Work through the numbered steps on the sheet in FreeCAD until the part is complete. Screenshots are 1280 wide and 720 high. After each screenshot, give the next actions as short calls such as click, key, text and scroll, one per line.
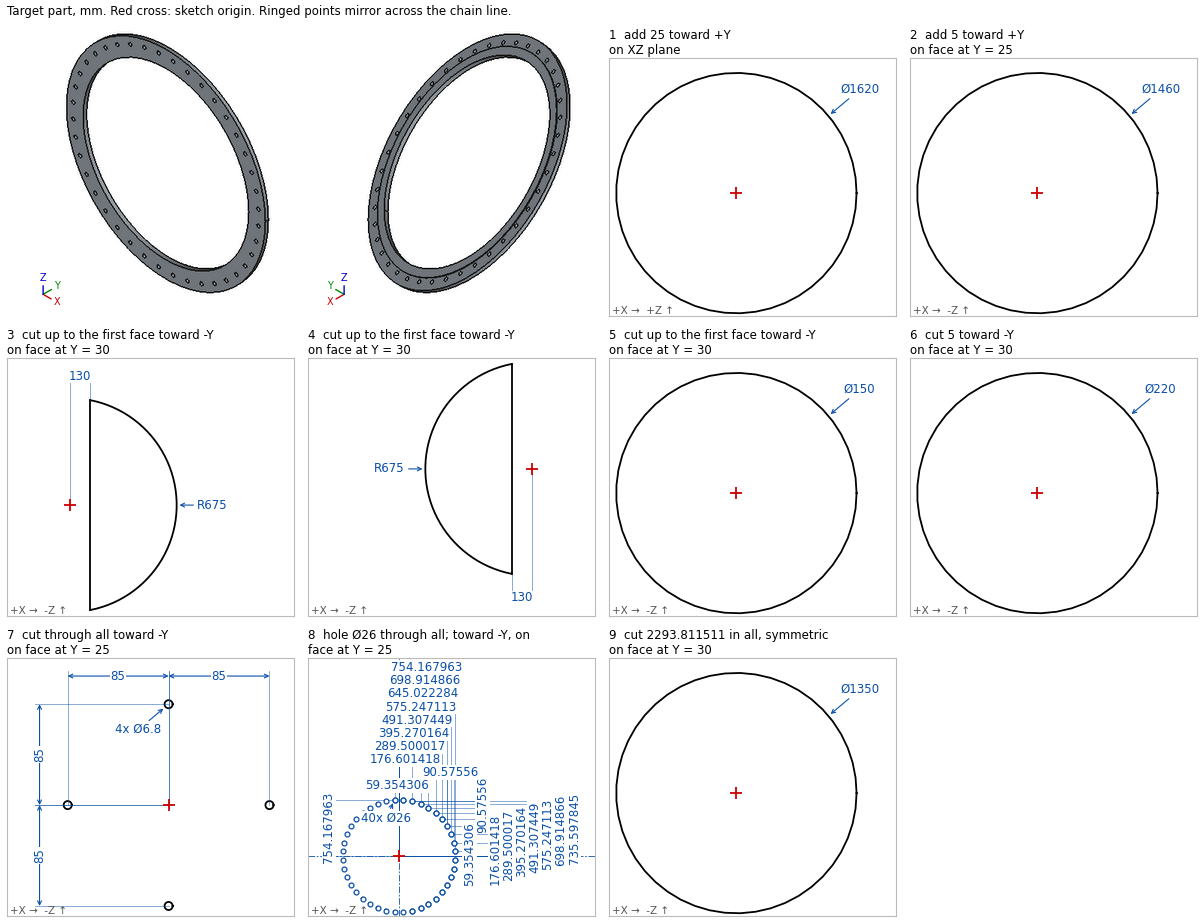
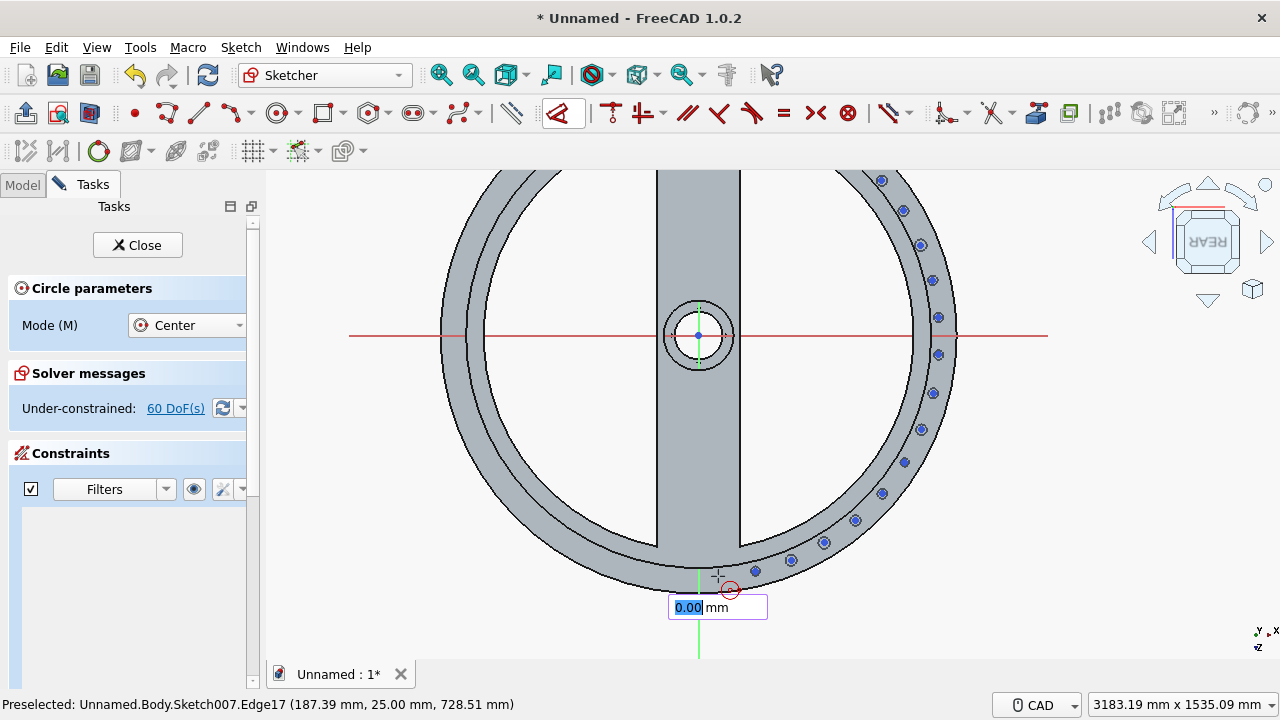
scroll(720, 573, up, 7)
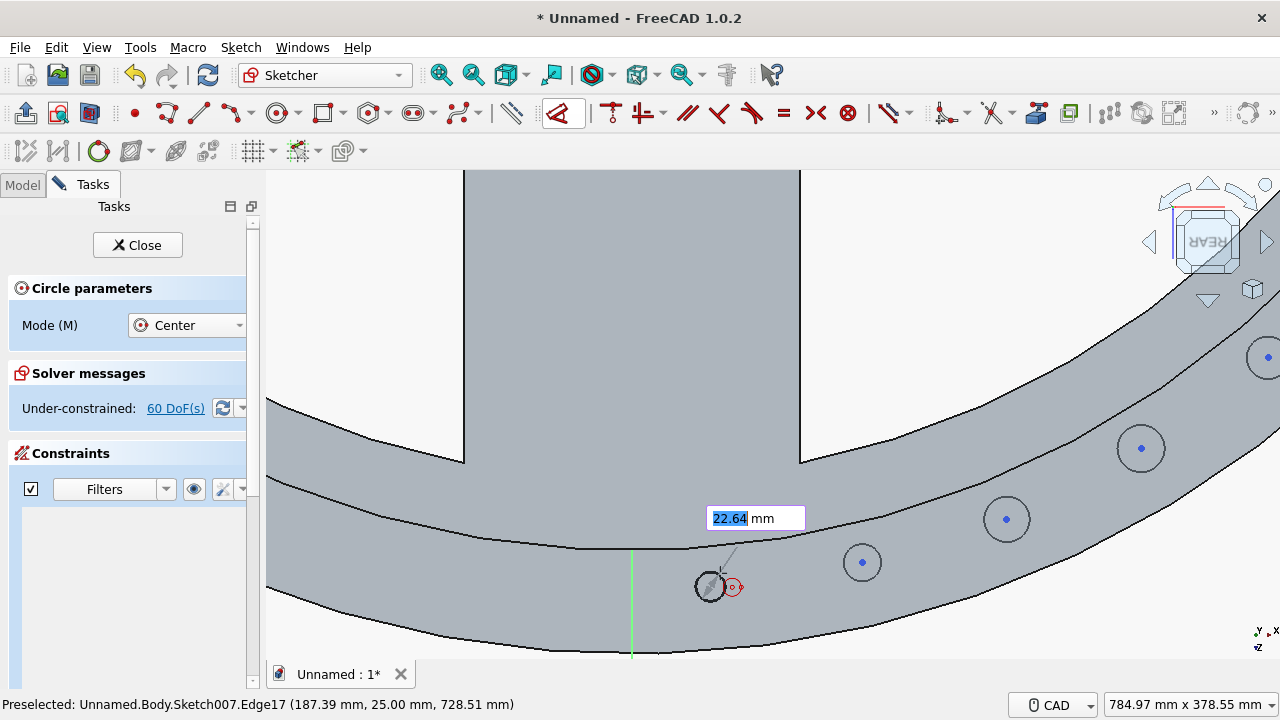
click(721, 570)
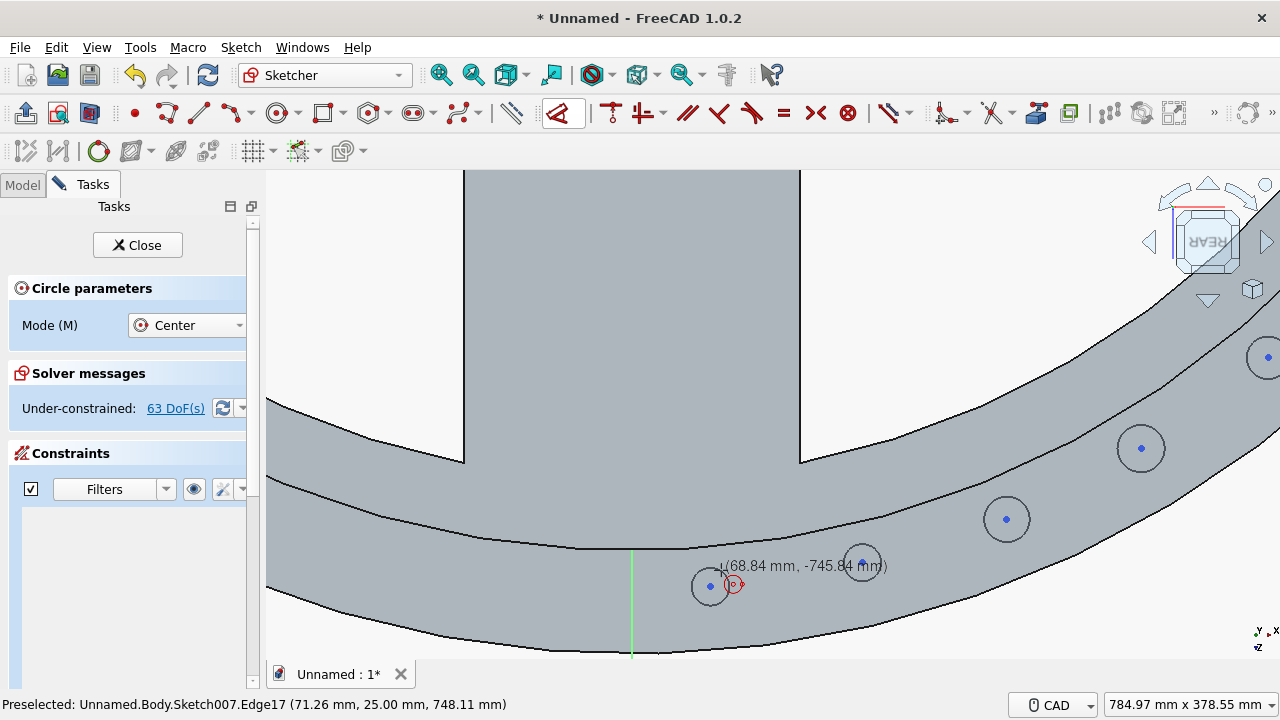
scroll(555, 582, up, 2)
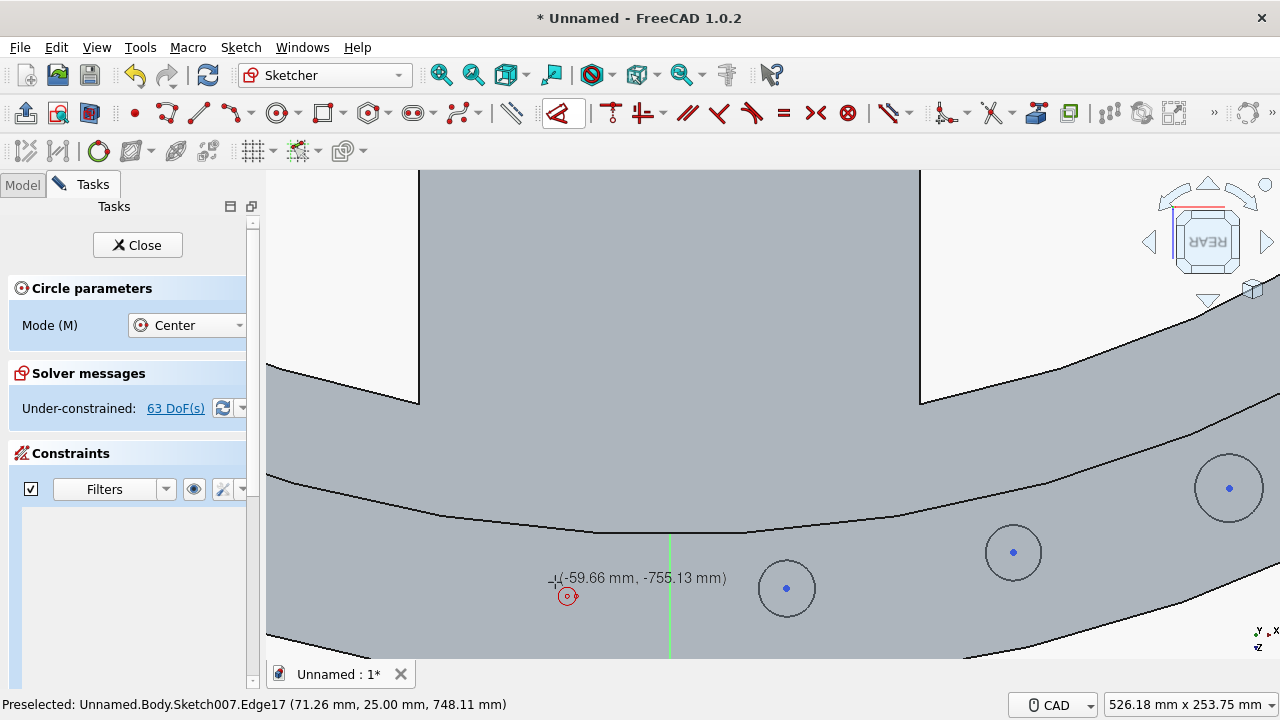
scroll(709, 575, down, 11)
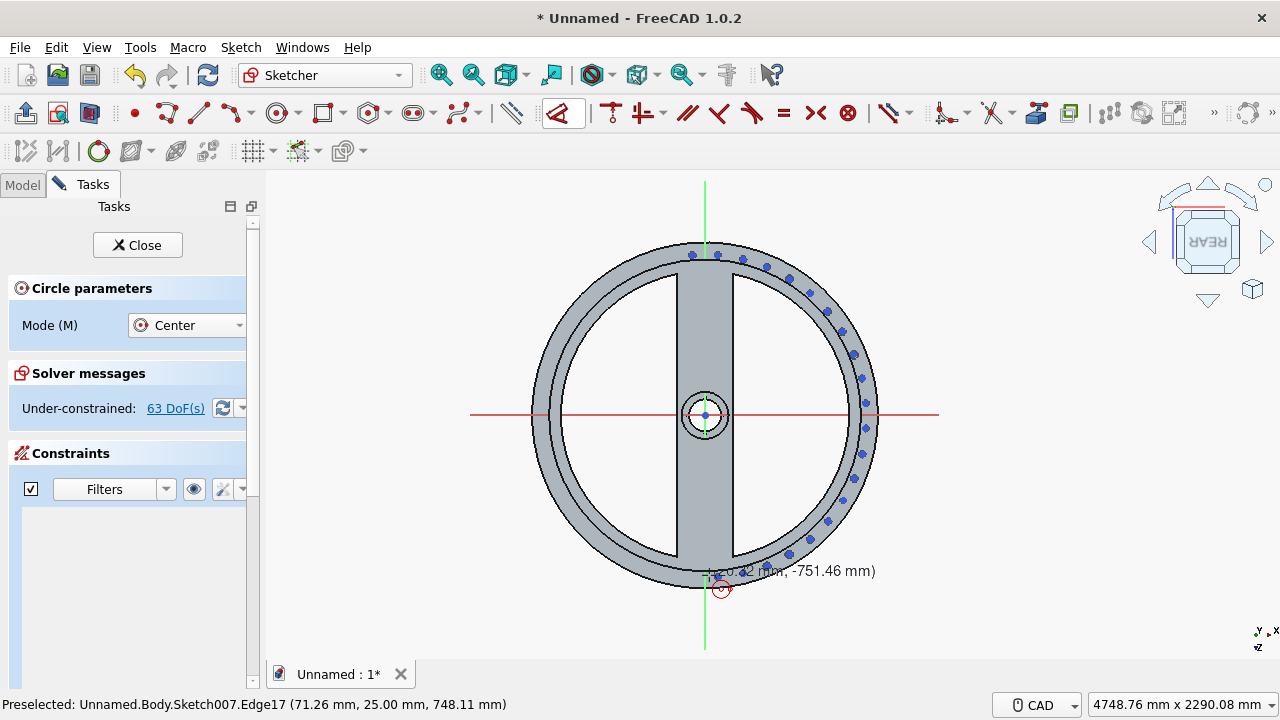
scroll(692, 576, up, 2)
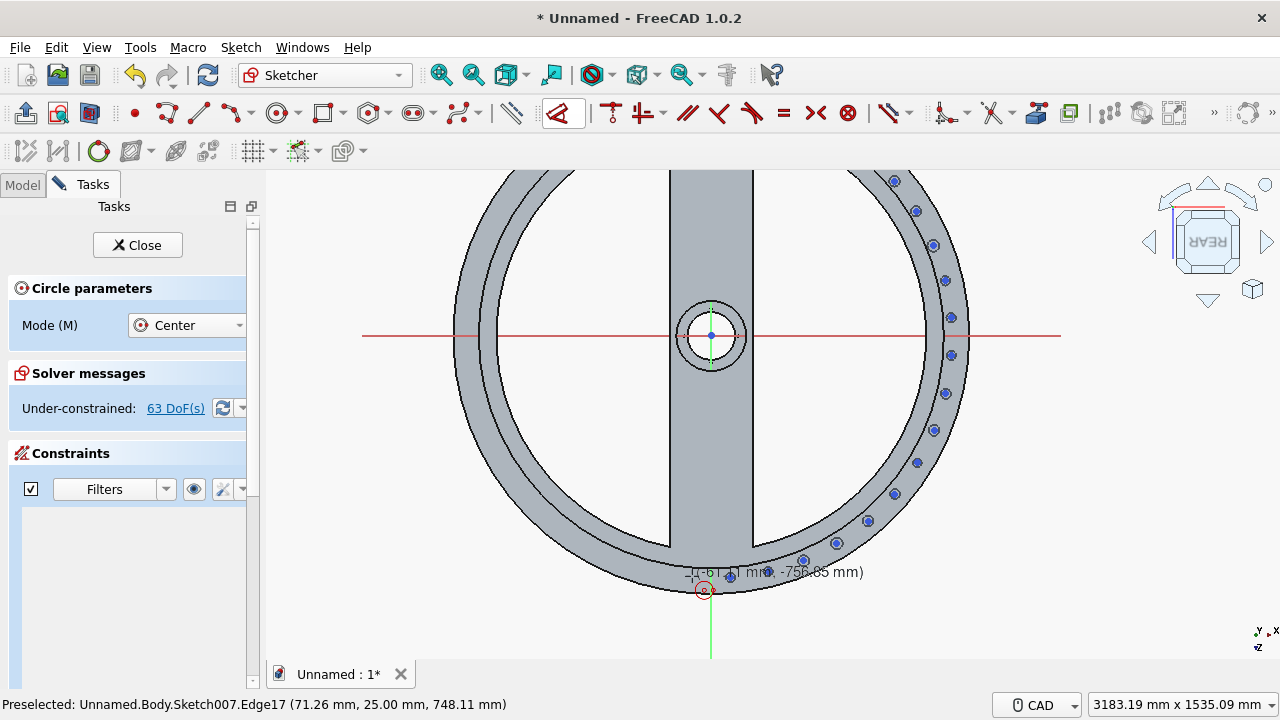
click(692, 576)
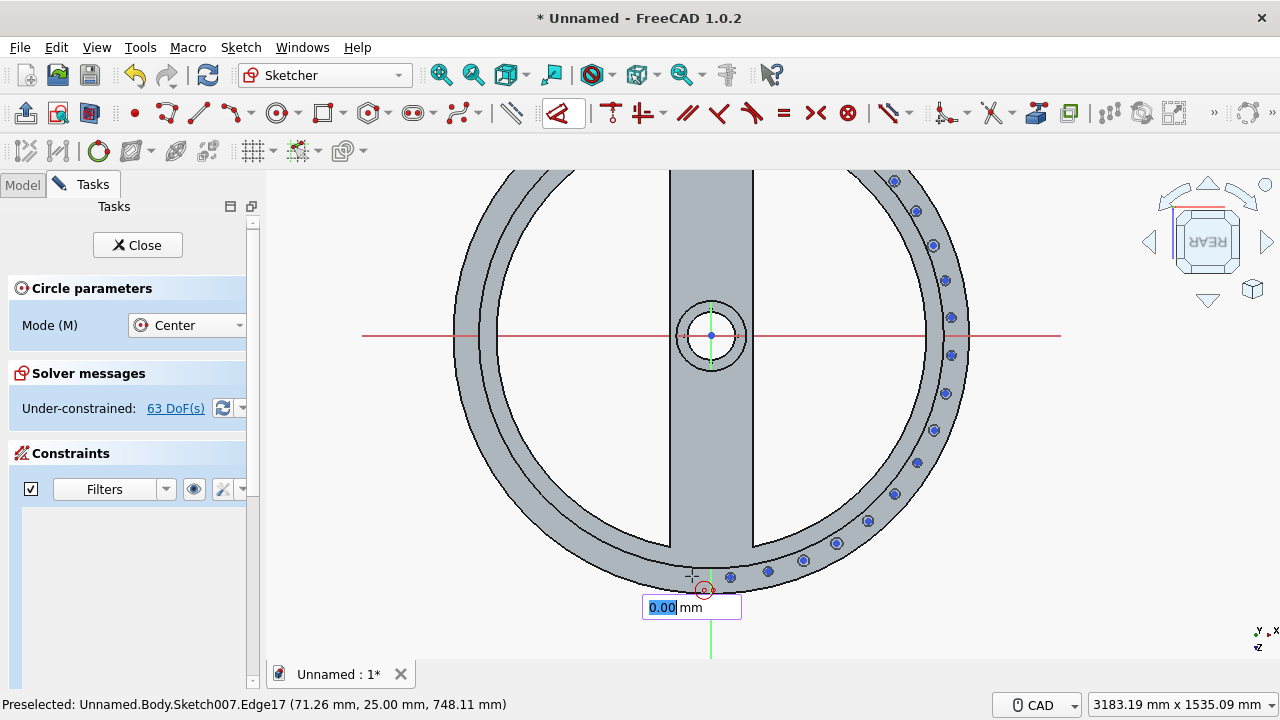
scroll(695, 573, up, 7)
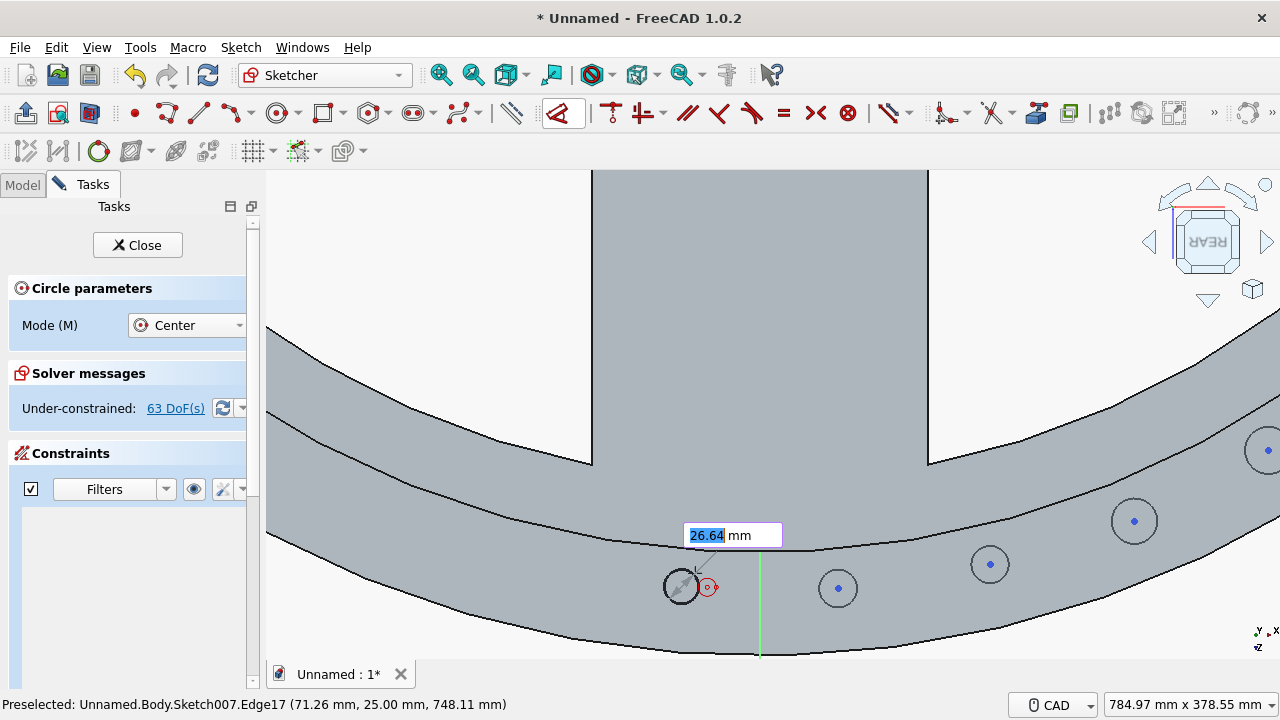
click(695, 572)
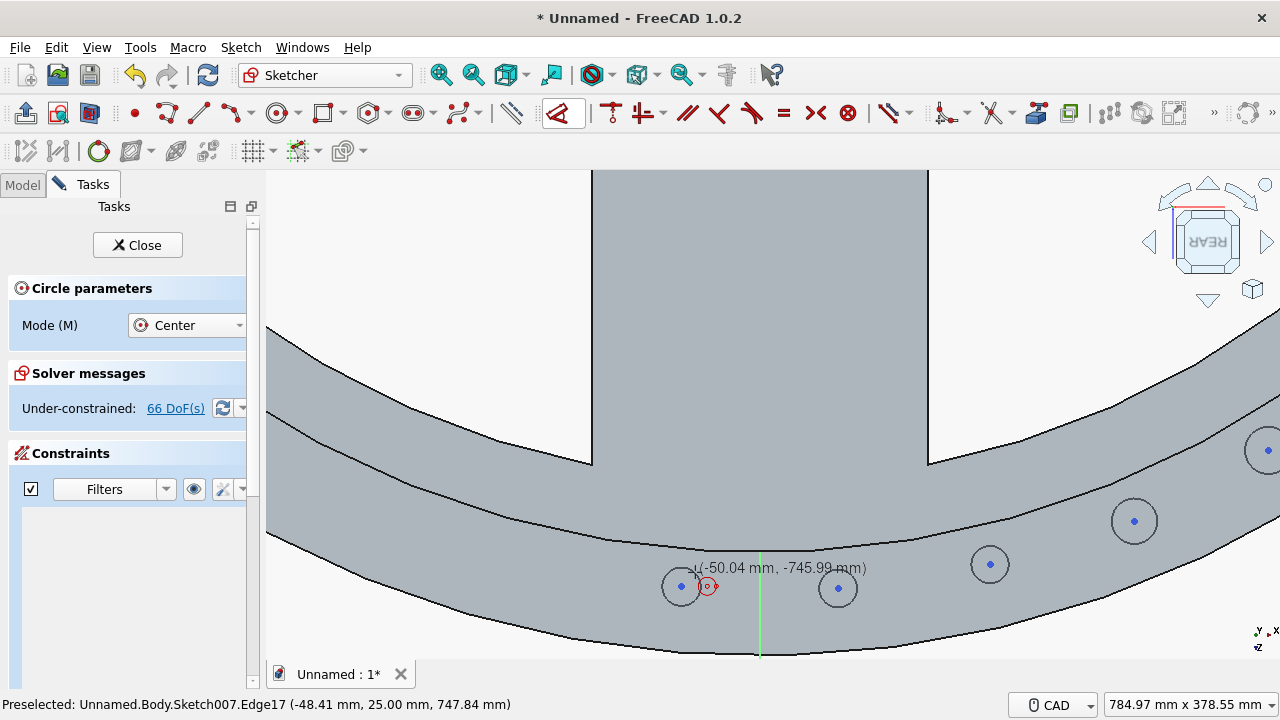
scroll(532, 560, up, 2)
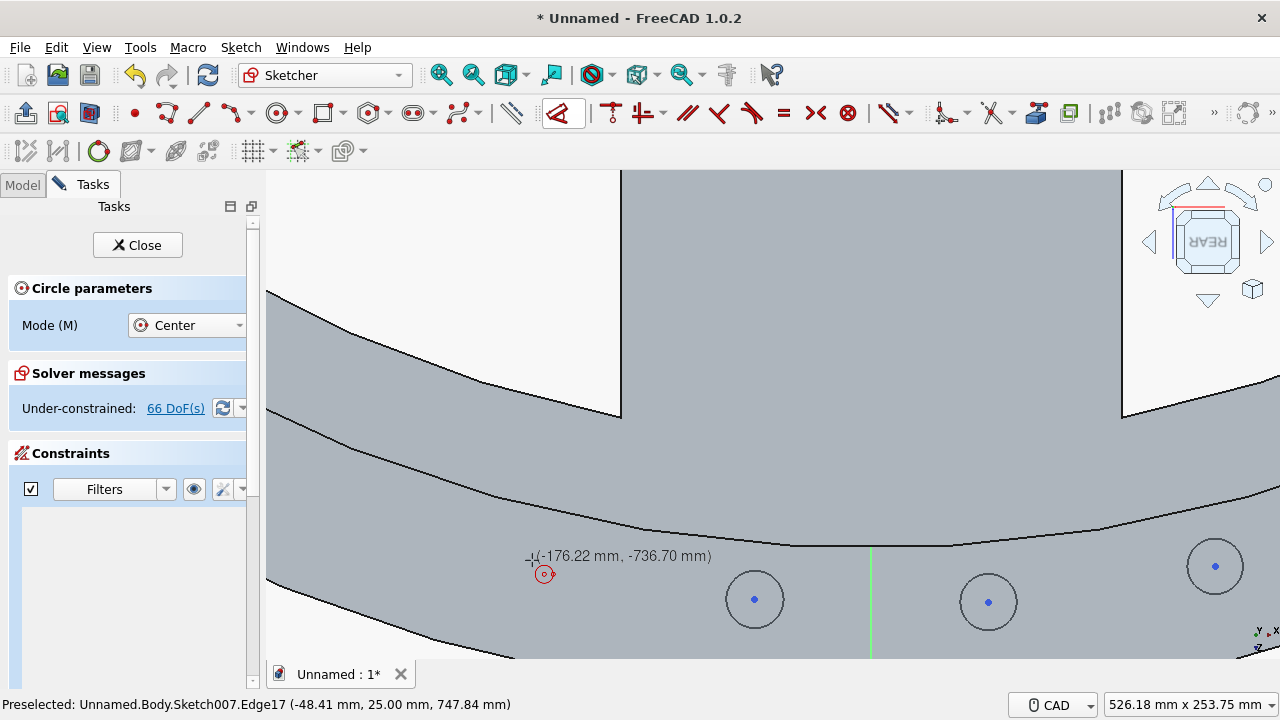
scroll(684, 573, down, 11)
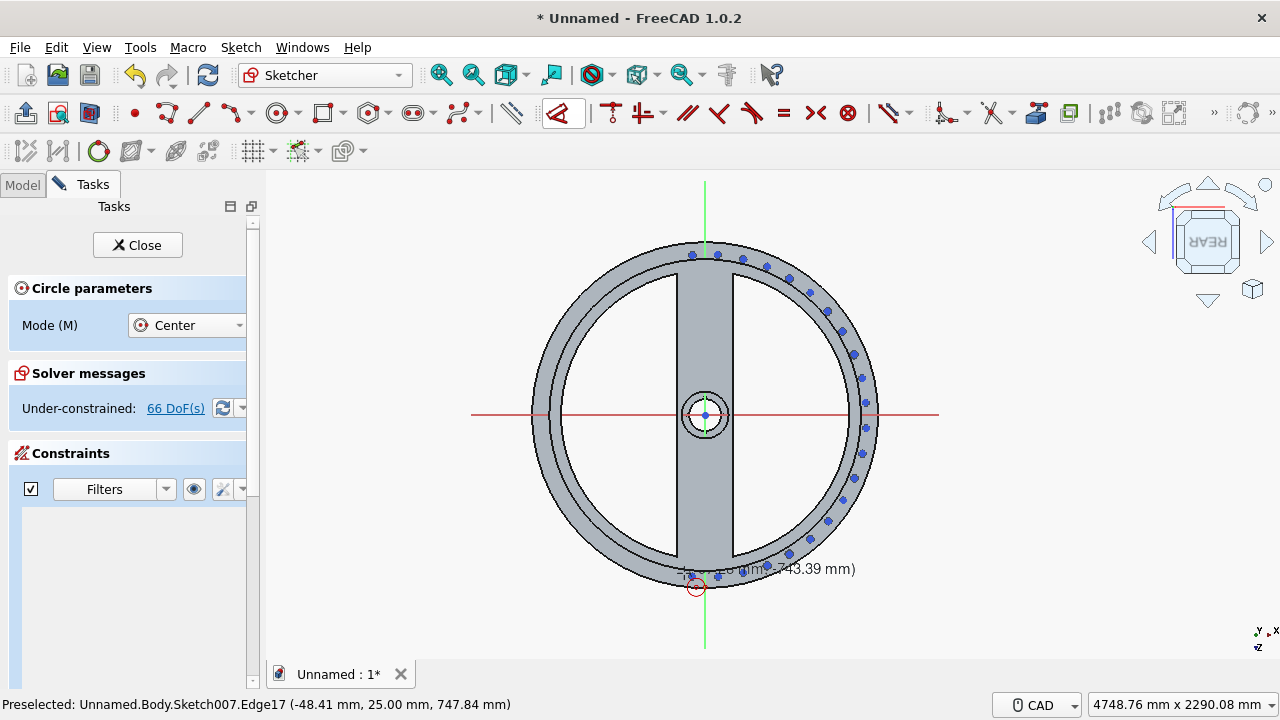
click(667, 572)